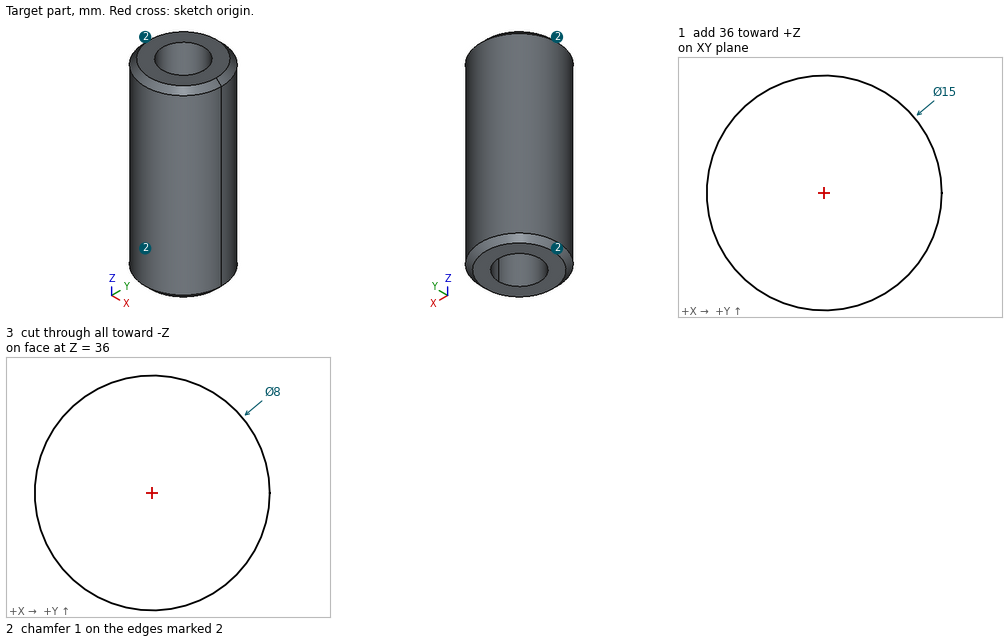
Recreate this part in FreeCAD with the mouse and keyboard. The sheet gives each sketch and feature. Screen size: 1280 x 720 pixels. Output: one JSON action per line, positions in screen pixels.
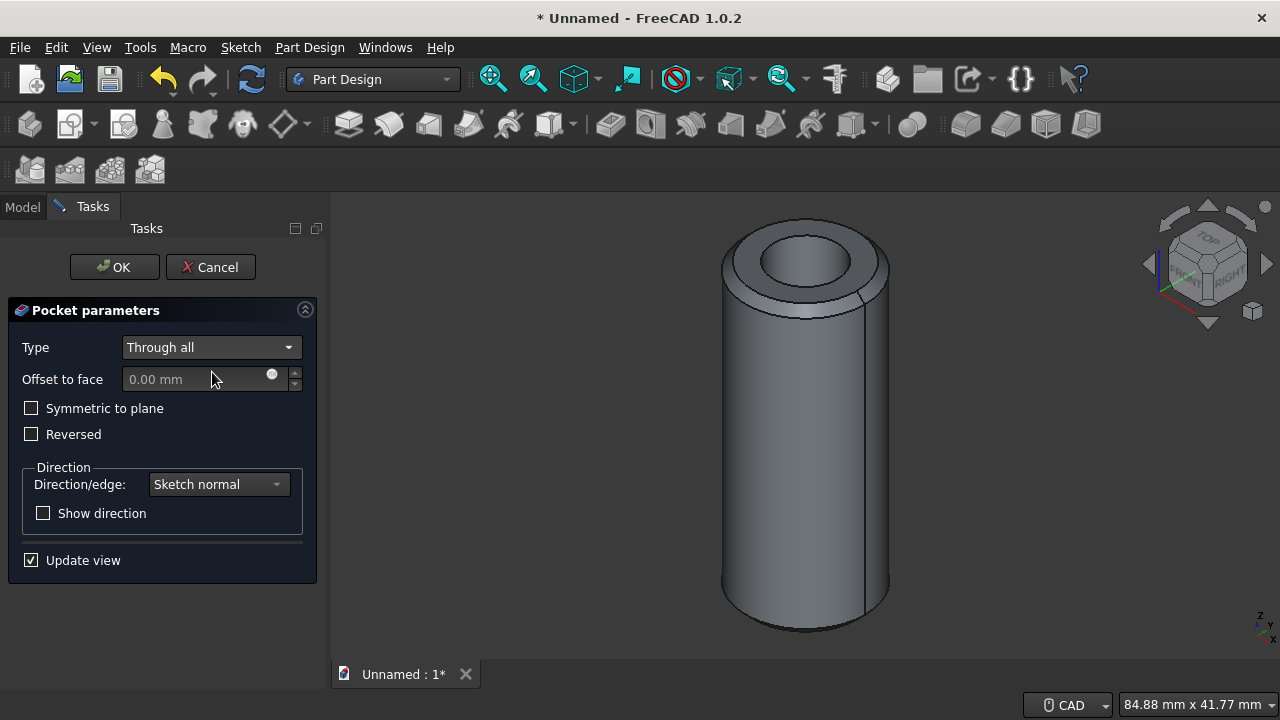
{"action": "left_click", "coordinate": [115, 267]}